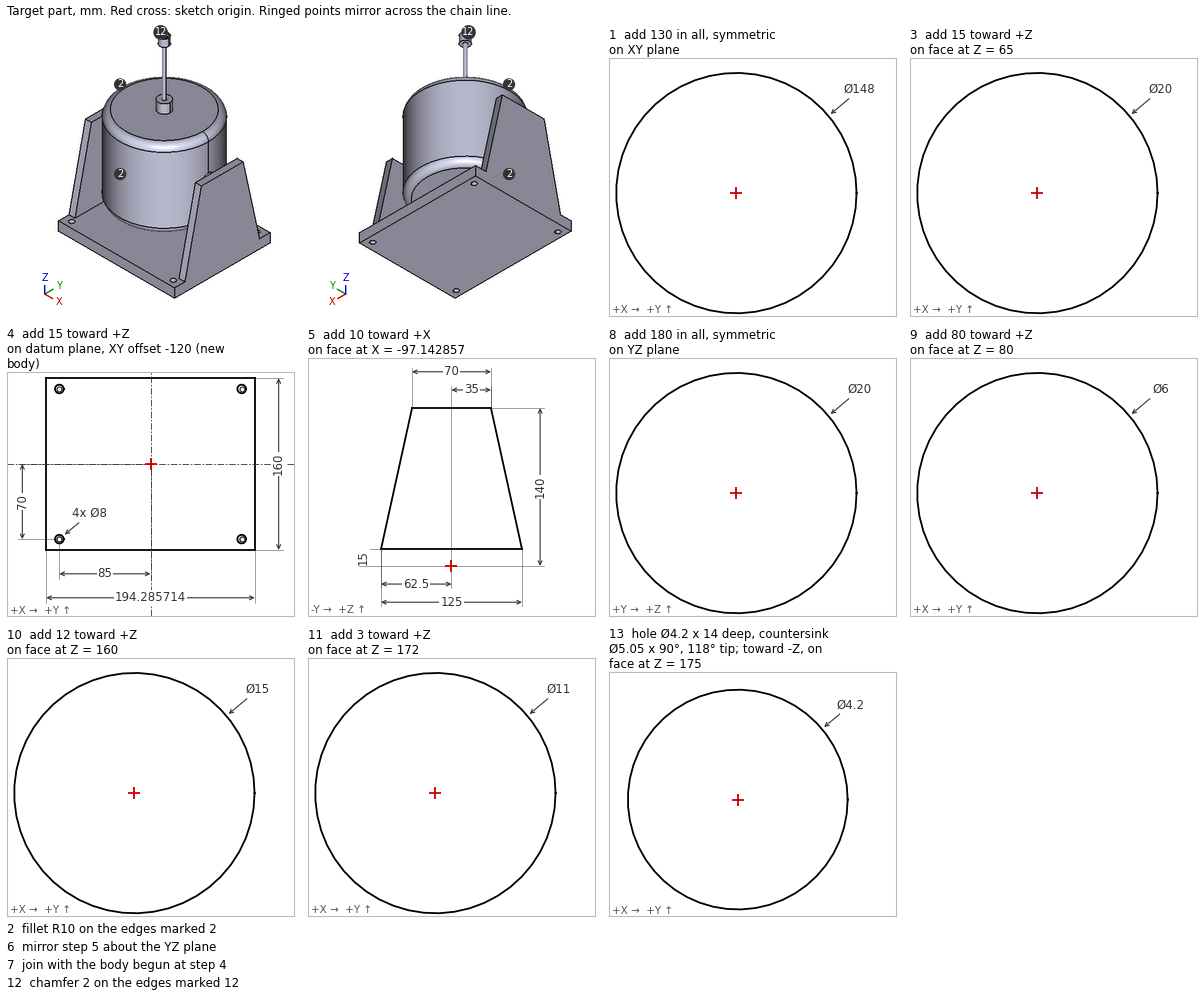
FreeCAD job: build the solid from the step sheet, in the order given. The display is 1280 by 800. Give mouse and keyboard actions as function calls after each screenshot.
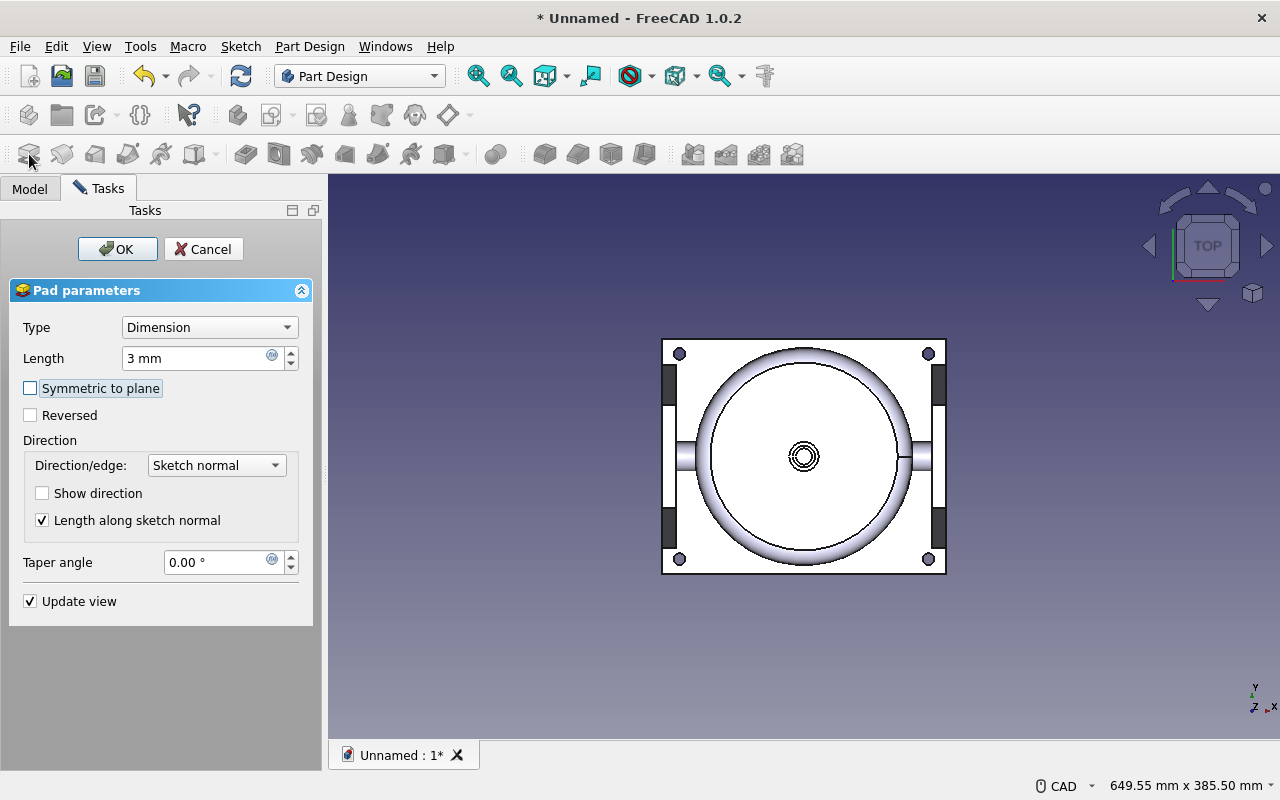
click(118, 249)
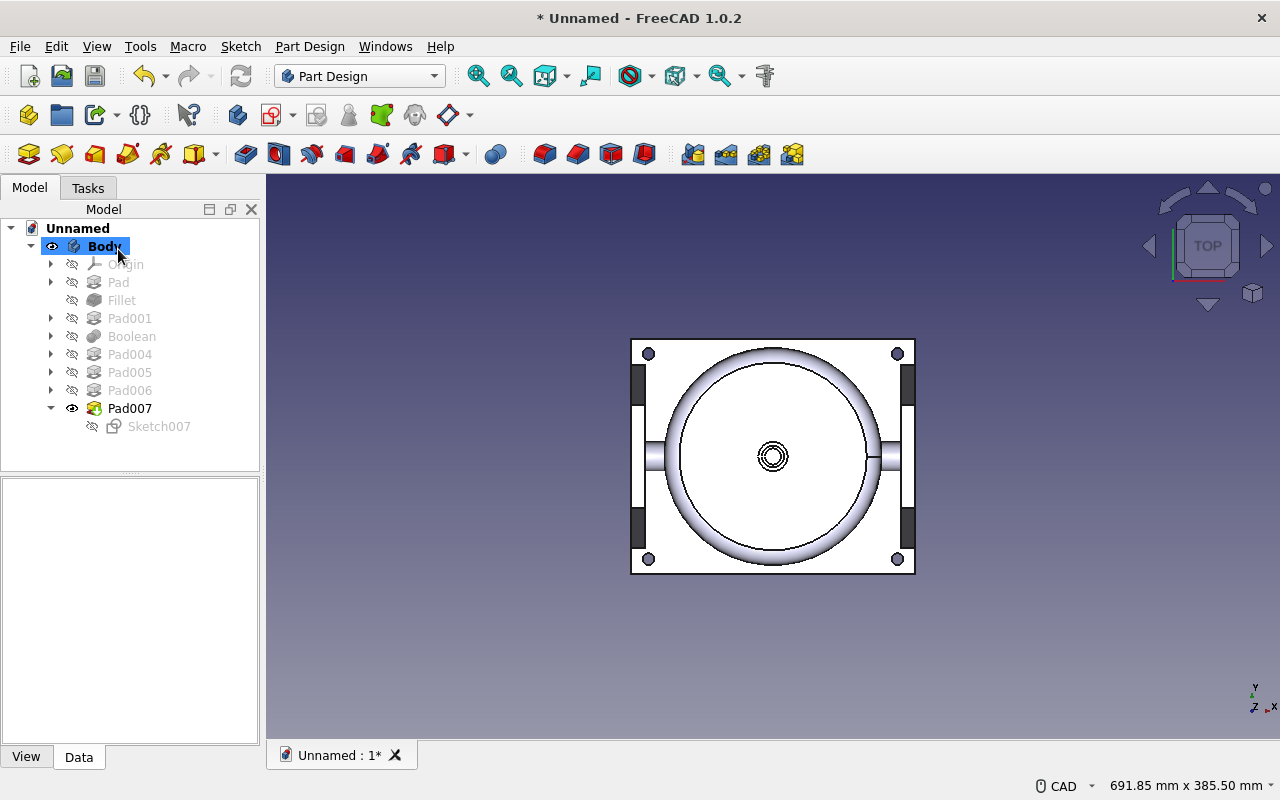
key(v)
key(f)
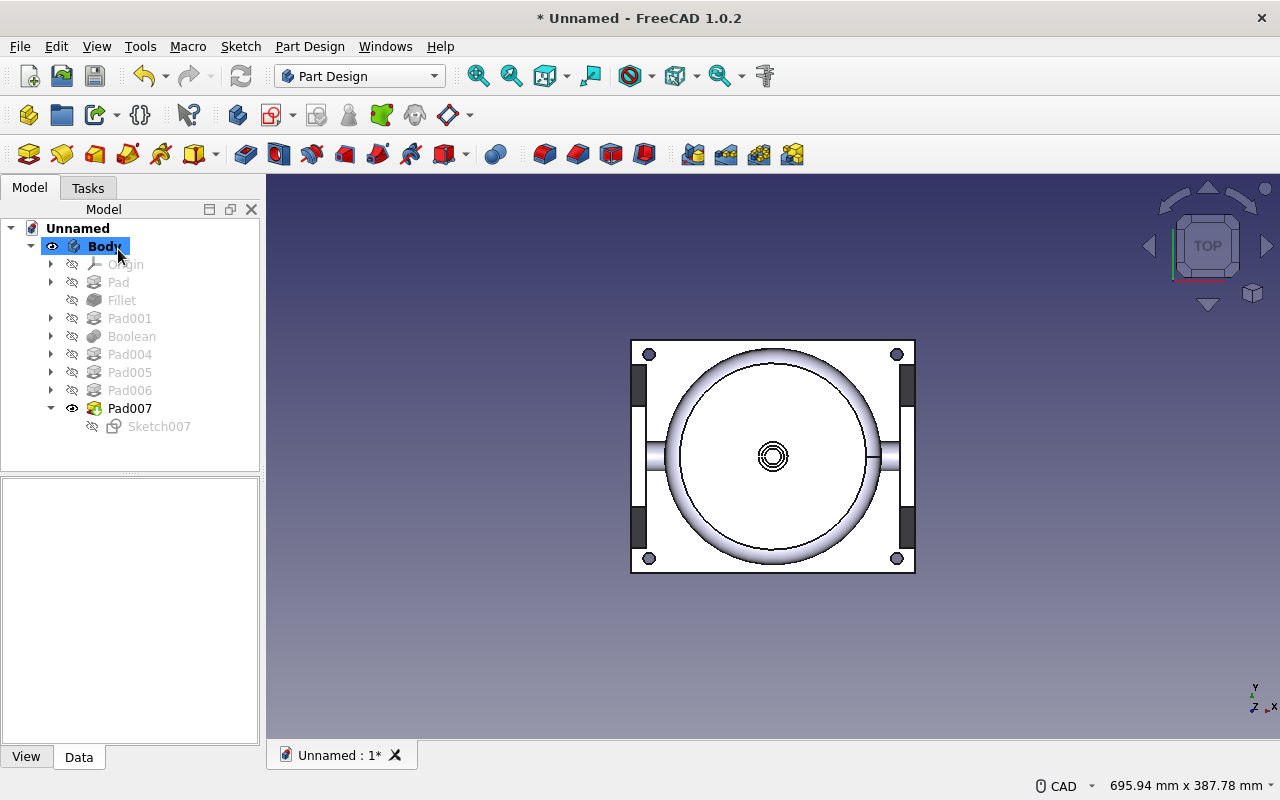
click(765, 455)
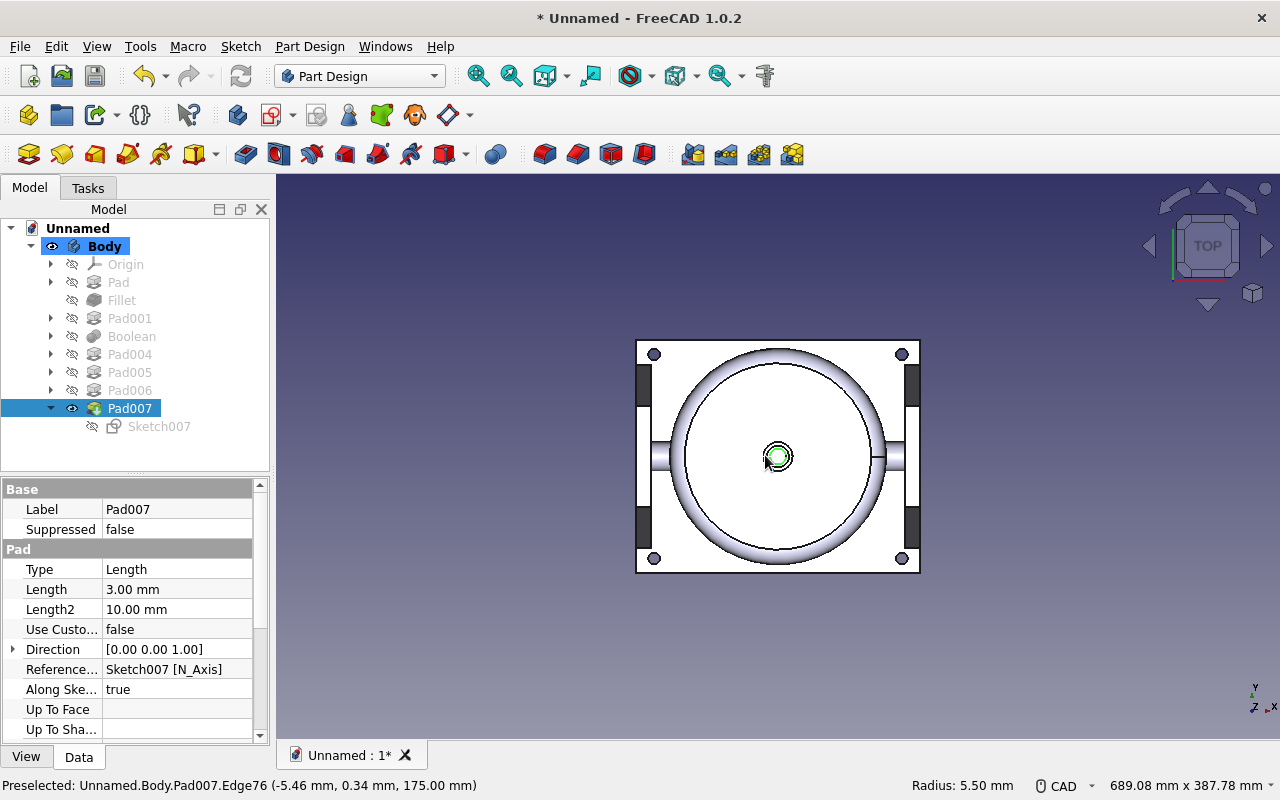
click(578, 154)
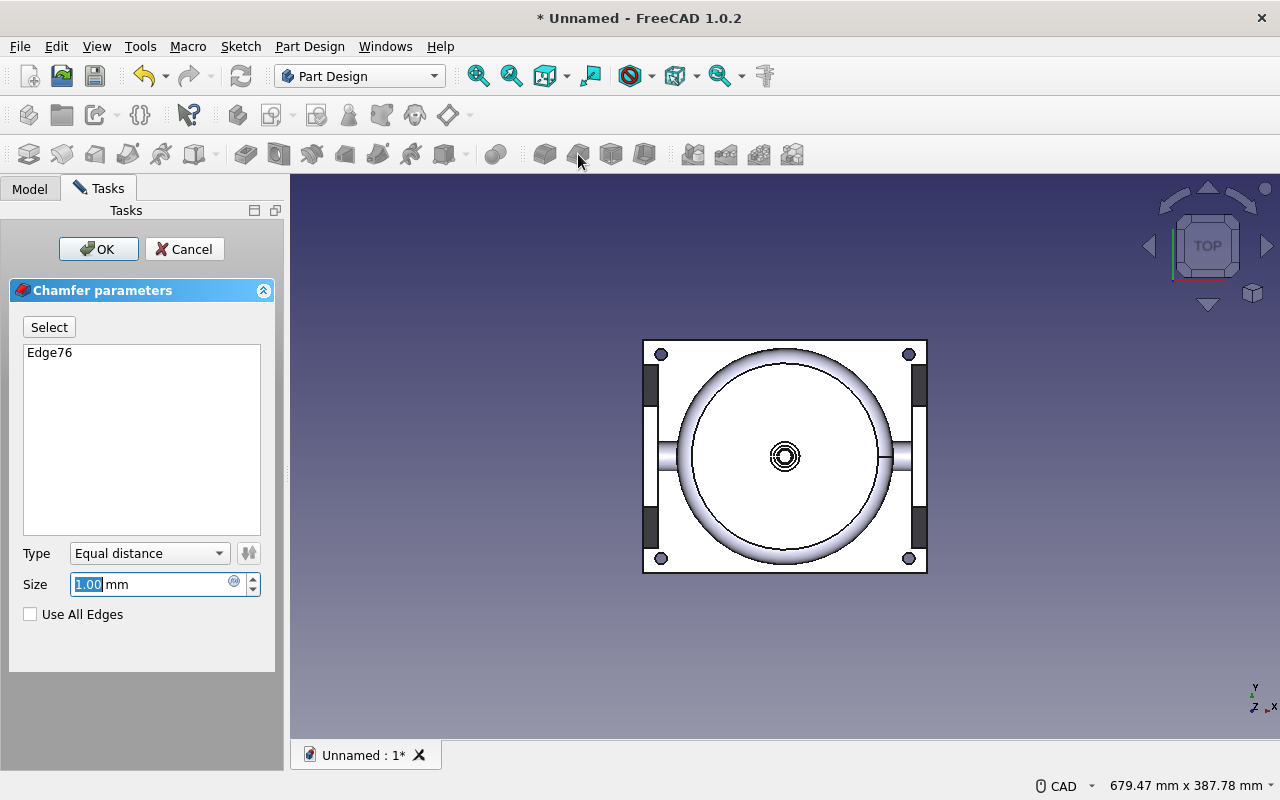
text(2)
key(Tab)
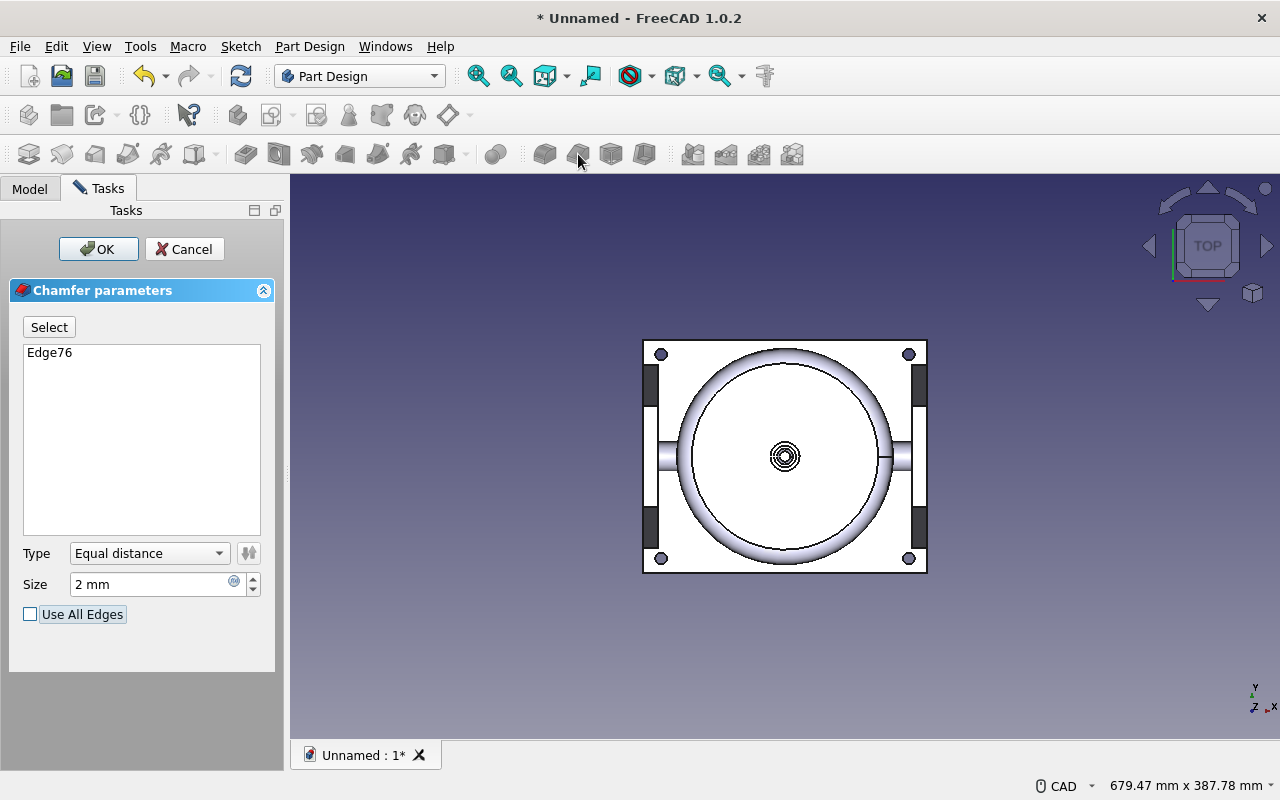
click(99, 249)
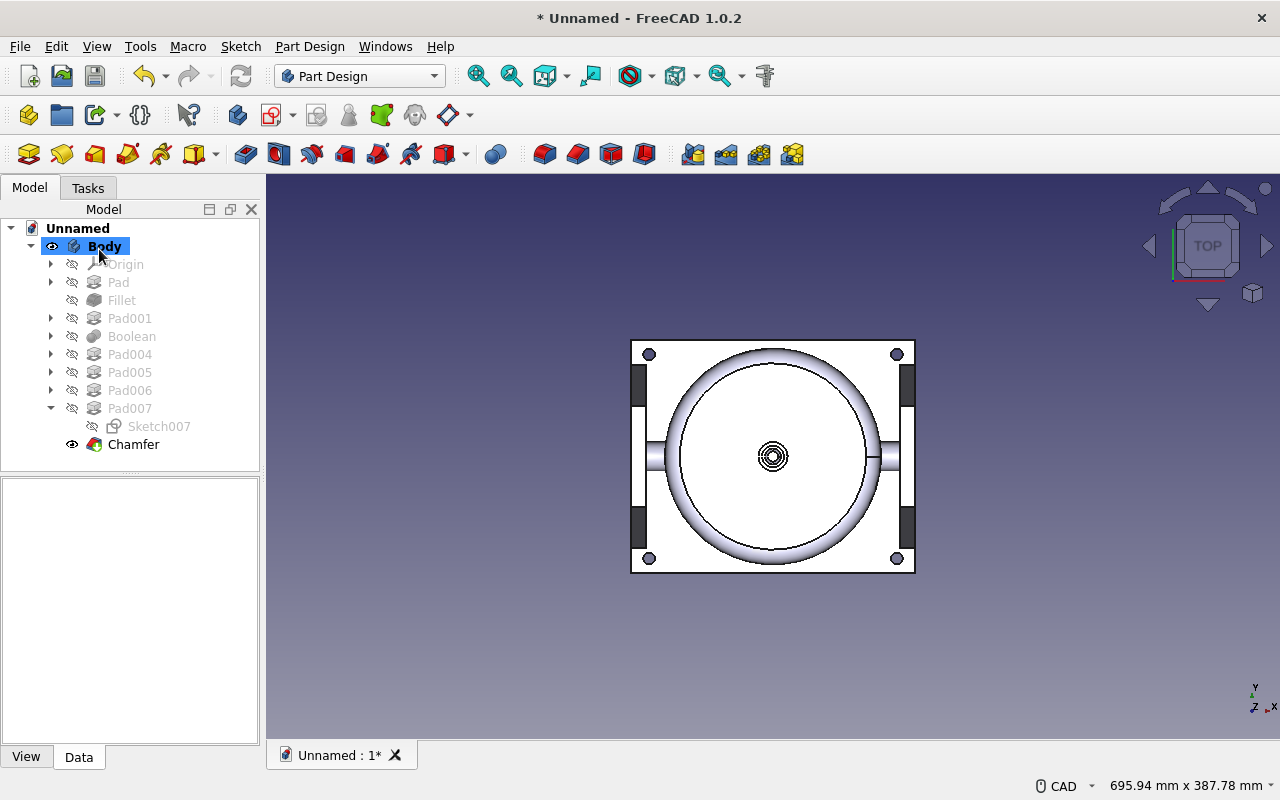
click(479, 76)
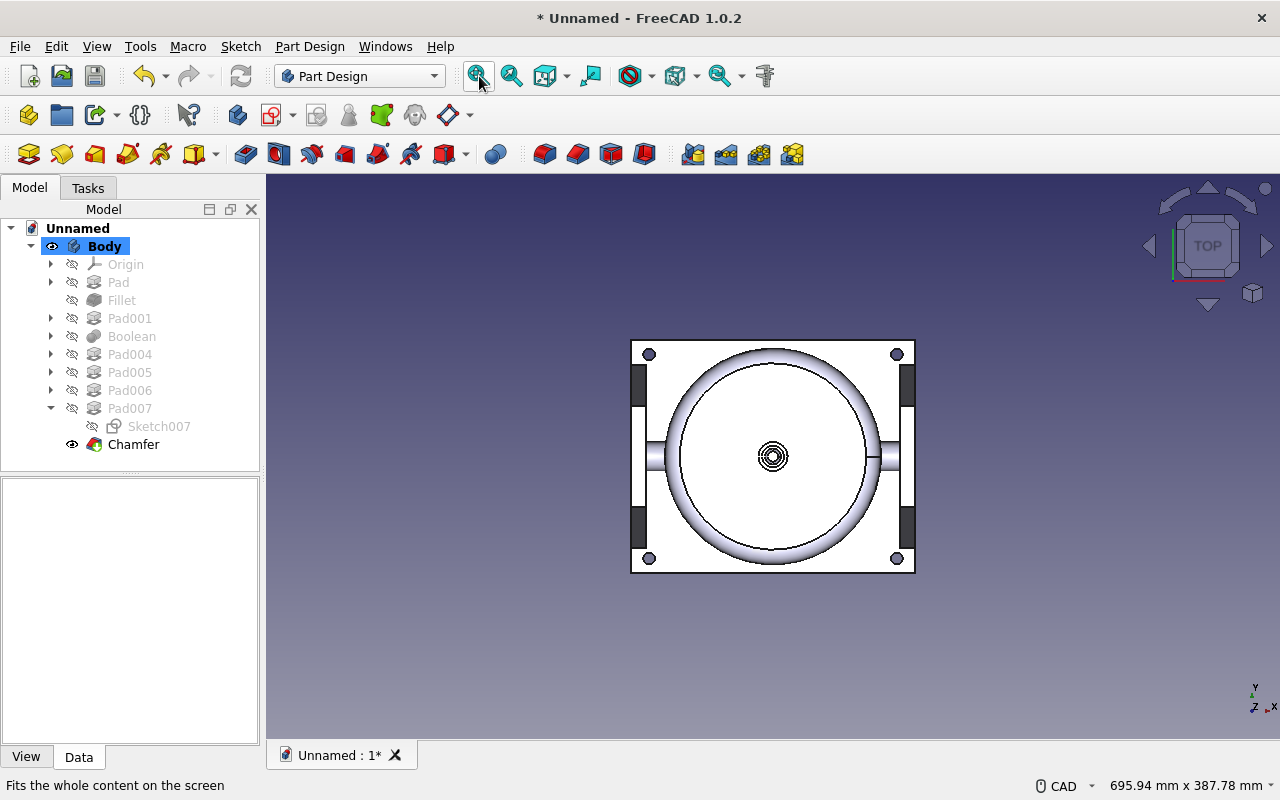
scroll(773, 455, up, 5)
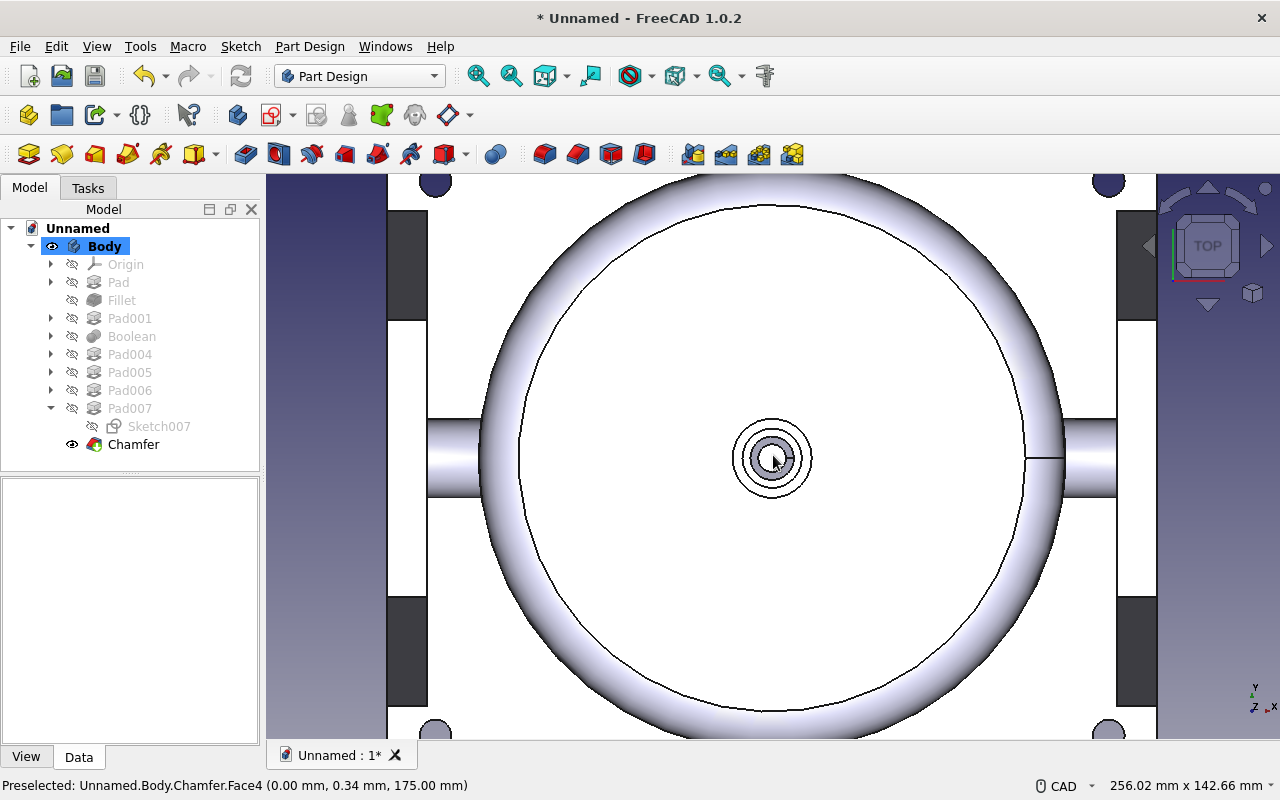
click(772, 457)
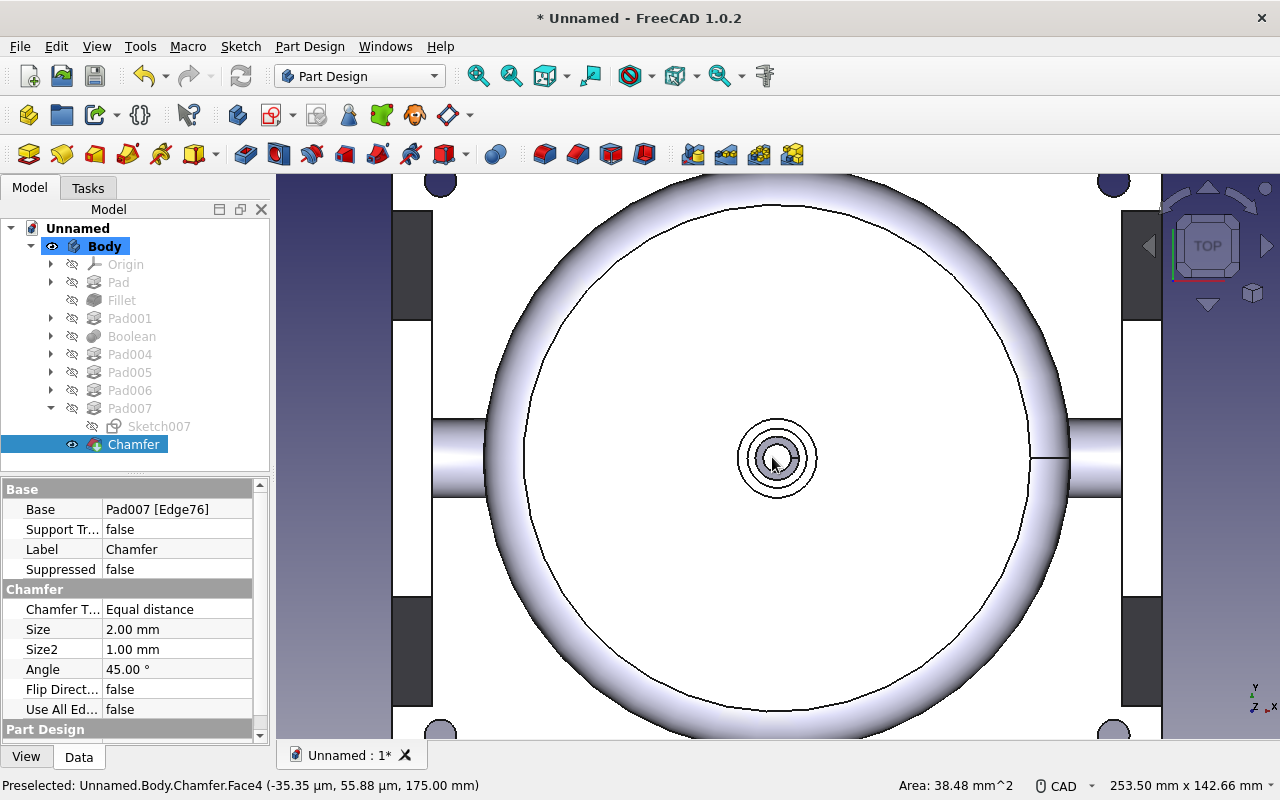
click(270, 116)